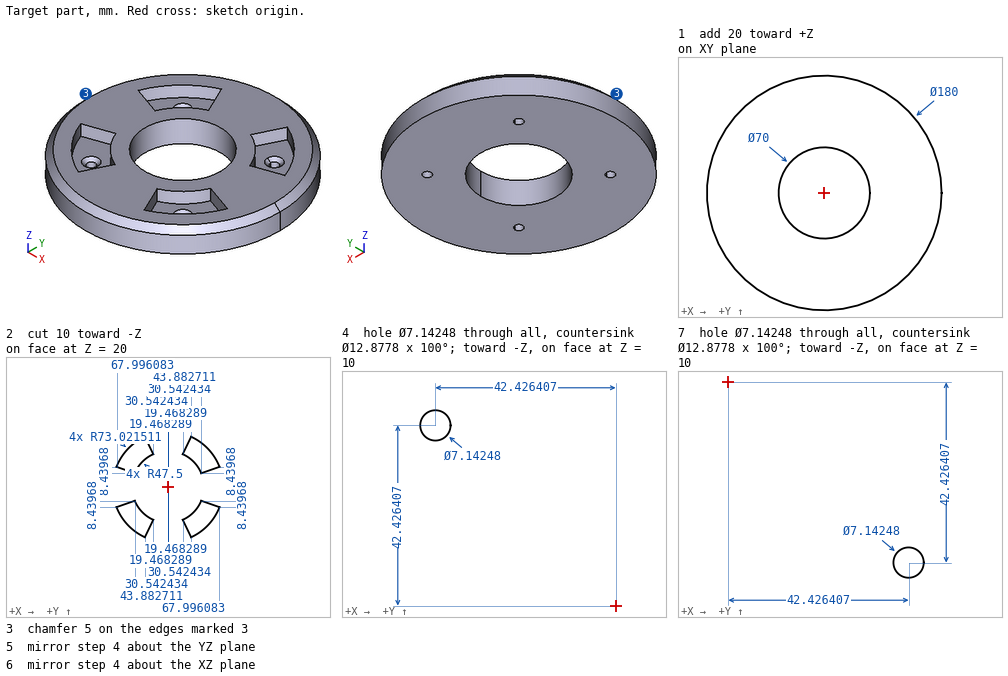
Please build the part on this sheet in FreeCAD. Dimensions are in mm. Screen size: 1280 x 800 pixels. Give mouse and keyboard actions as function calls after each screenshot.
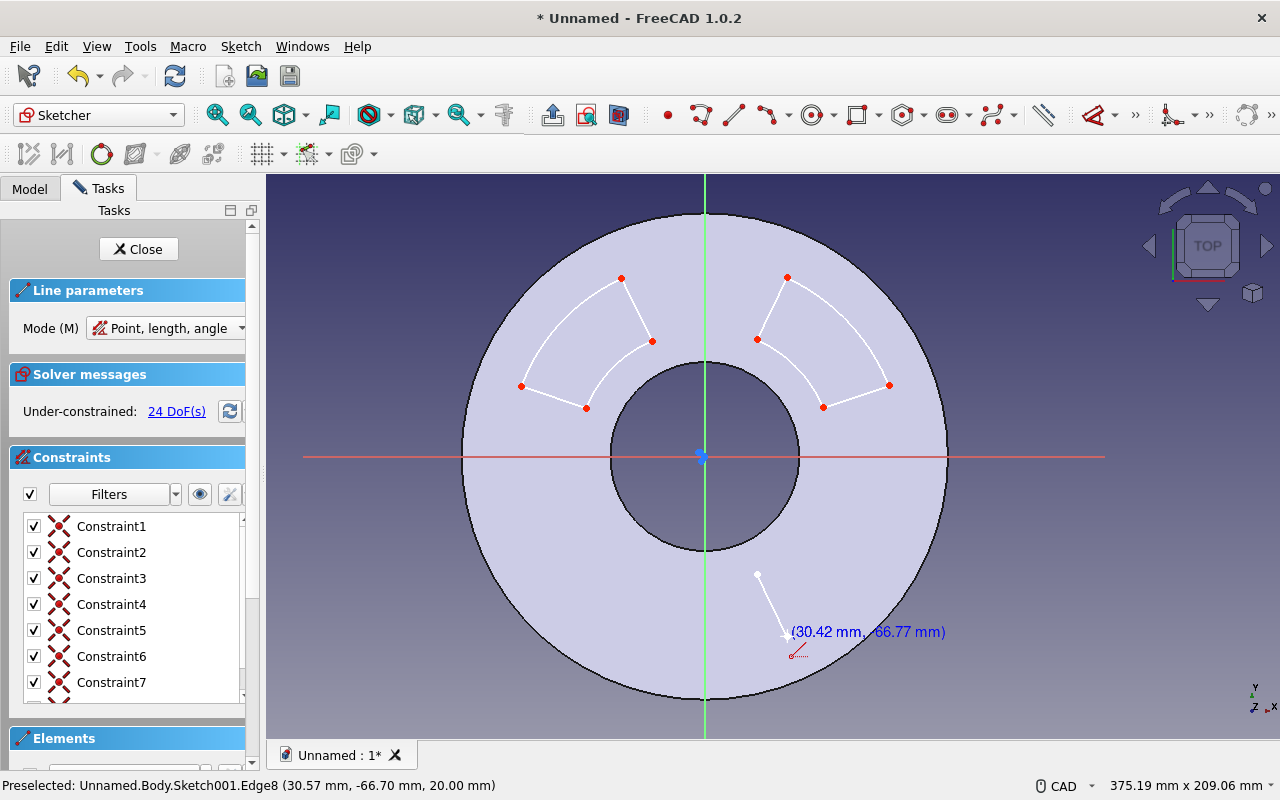
click(889, 528)
click(823, 506)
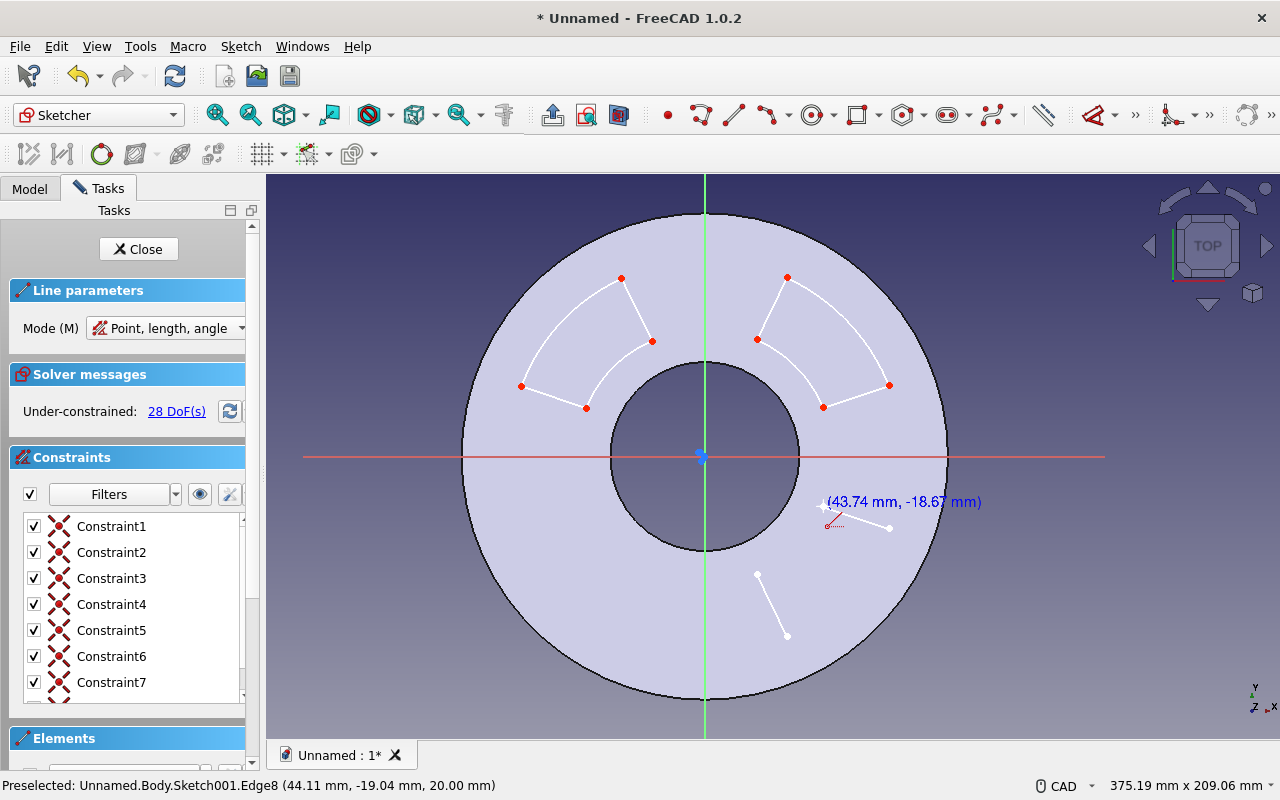
click(766, 116)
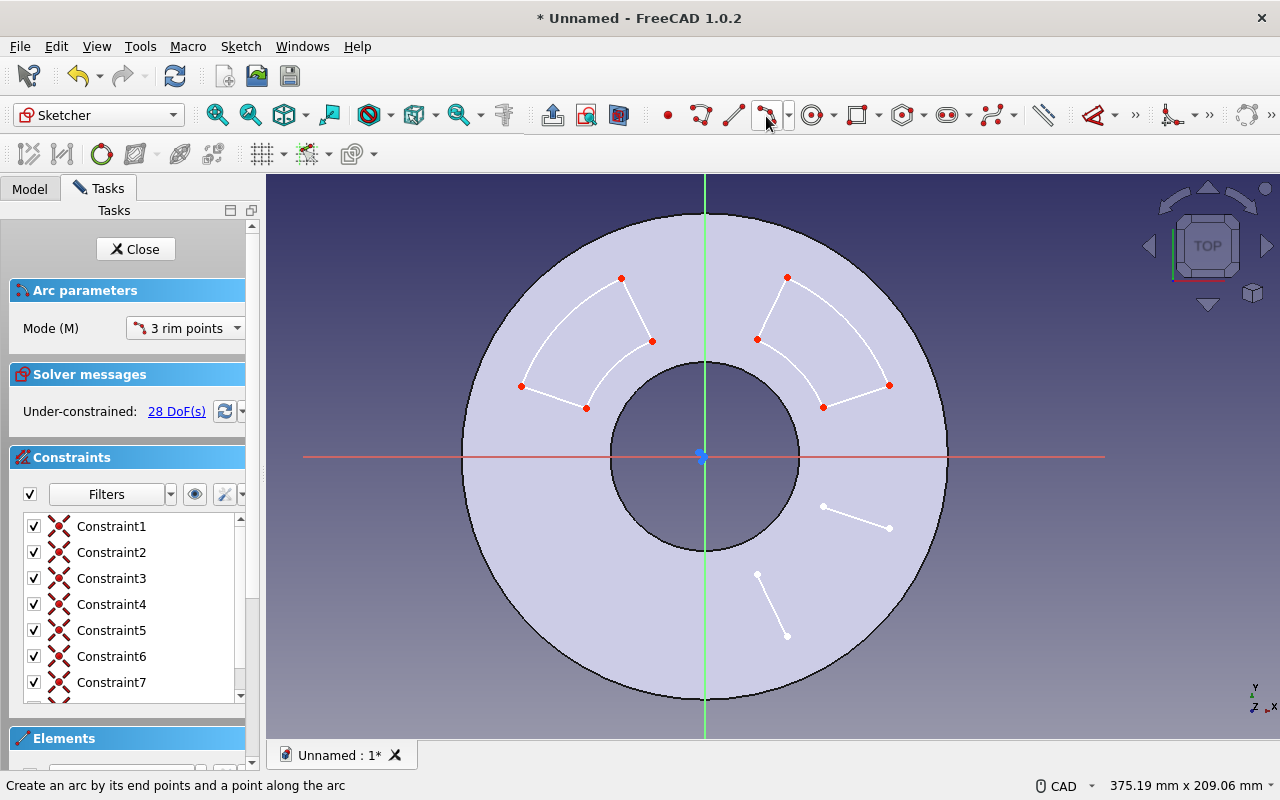
click(787, 637)
click(889, 529)
click(848, 592)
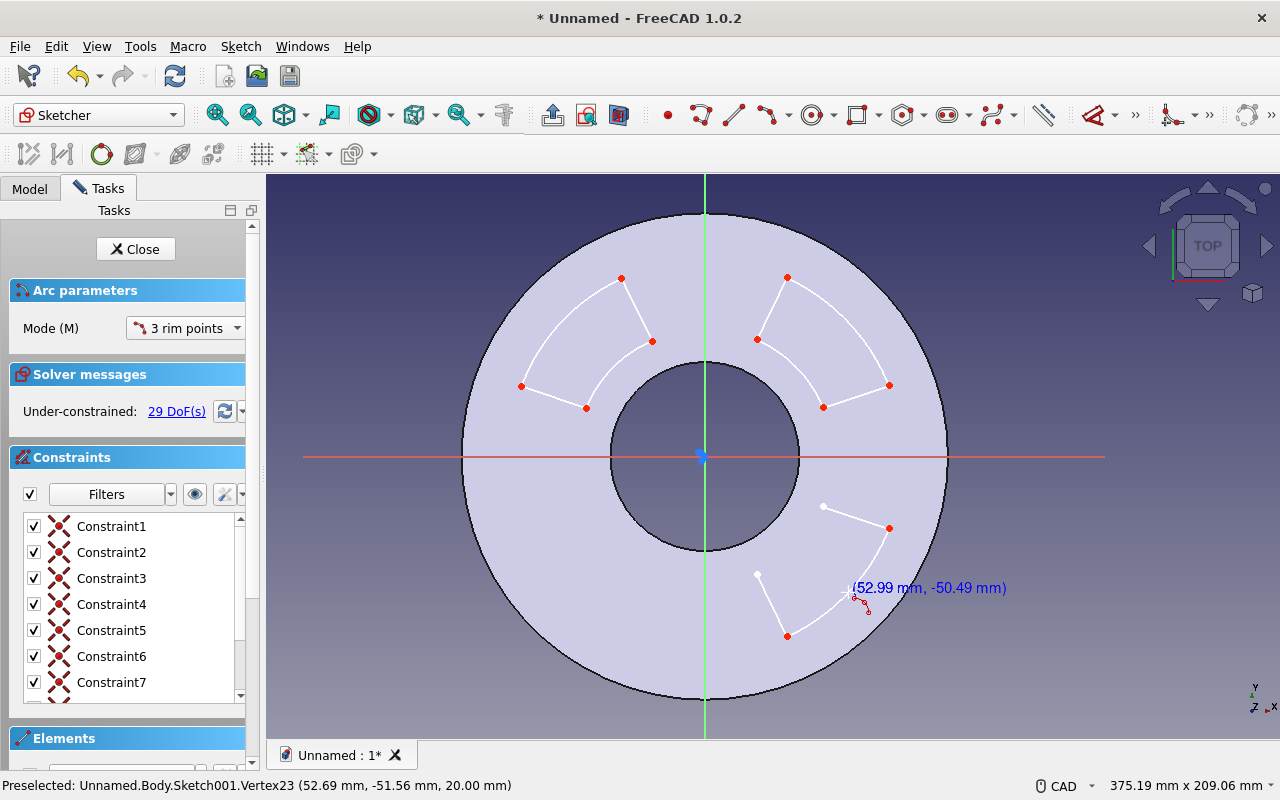
click(823, 507)
click(757, 575)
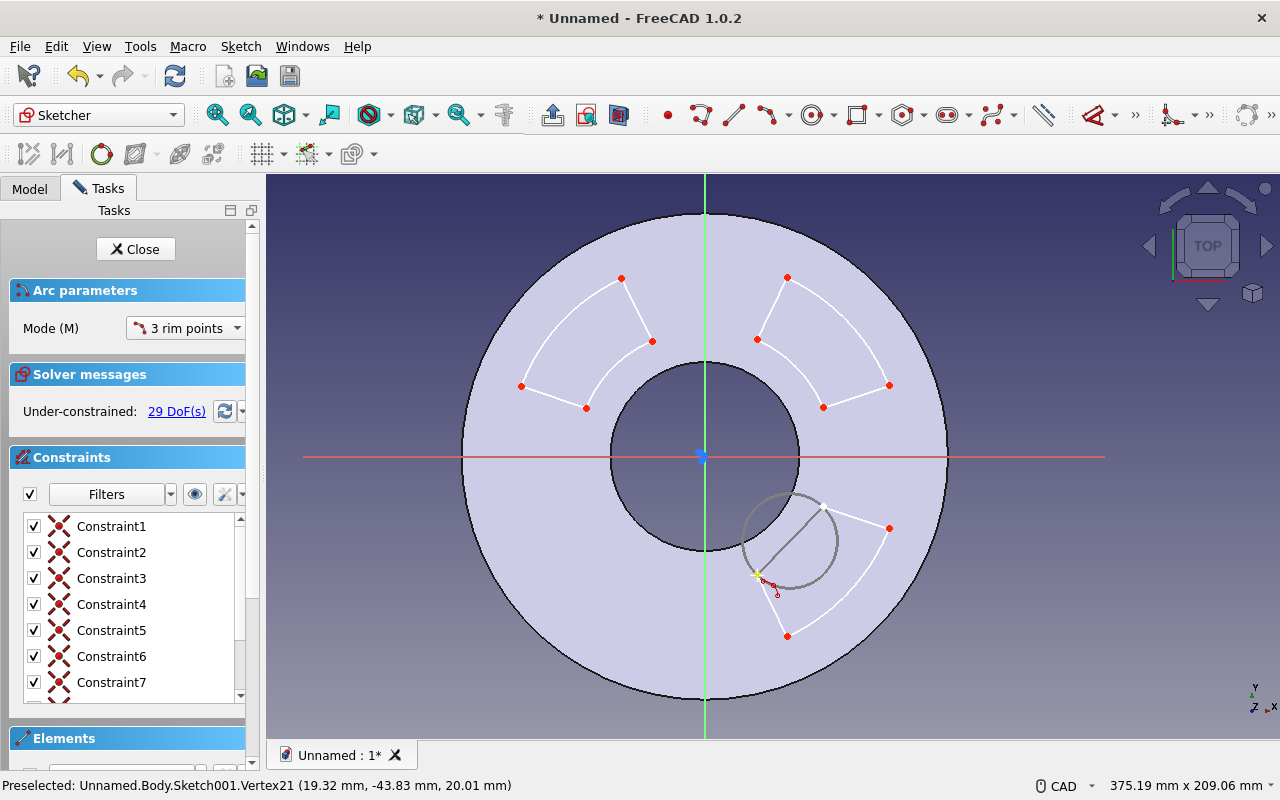
scroll(797, 546, up, 3)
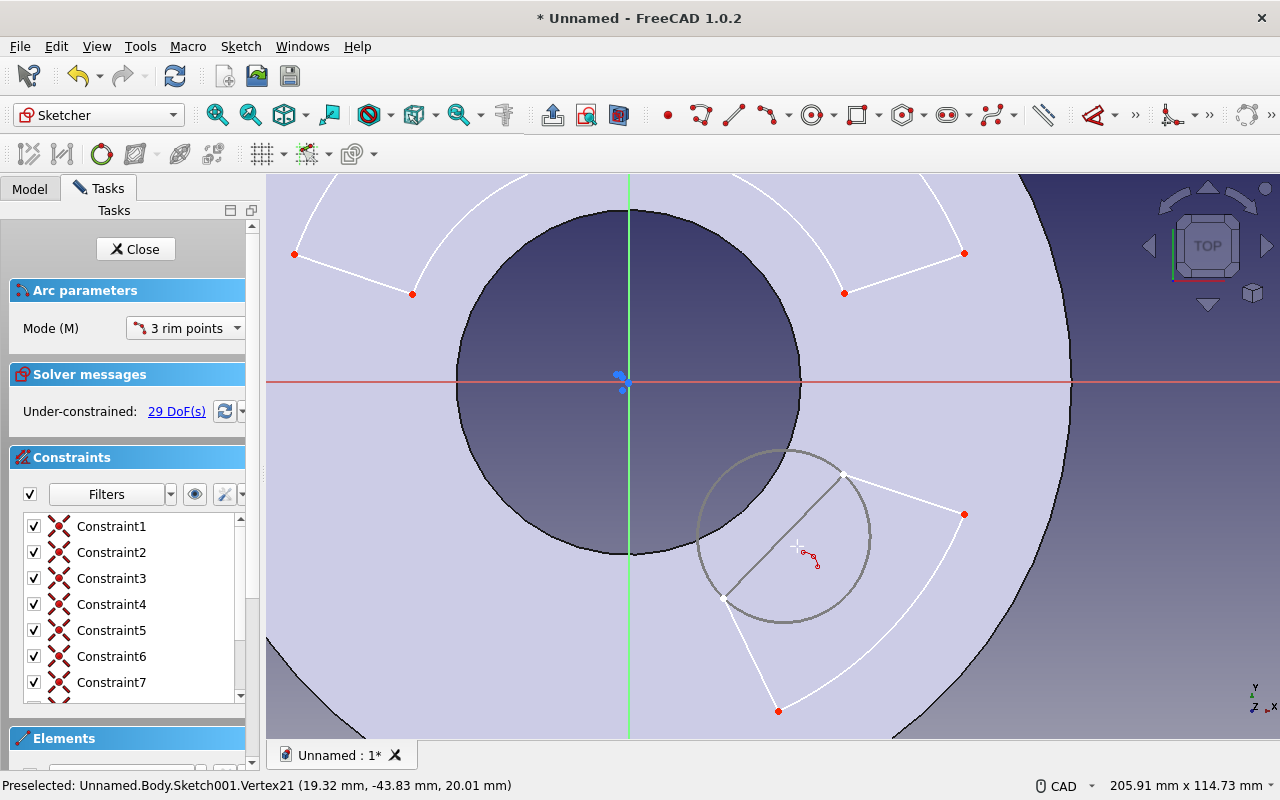
click(796, 545)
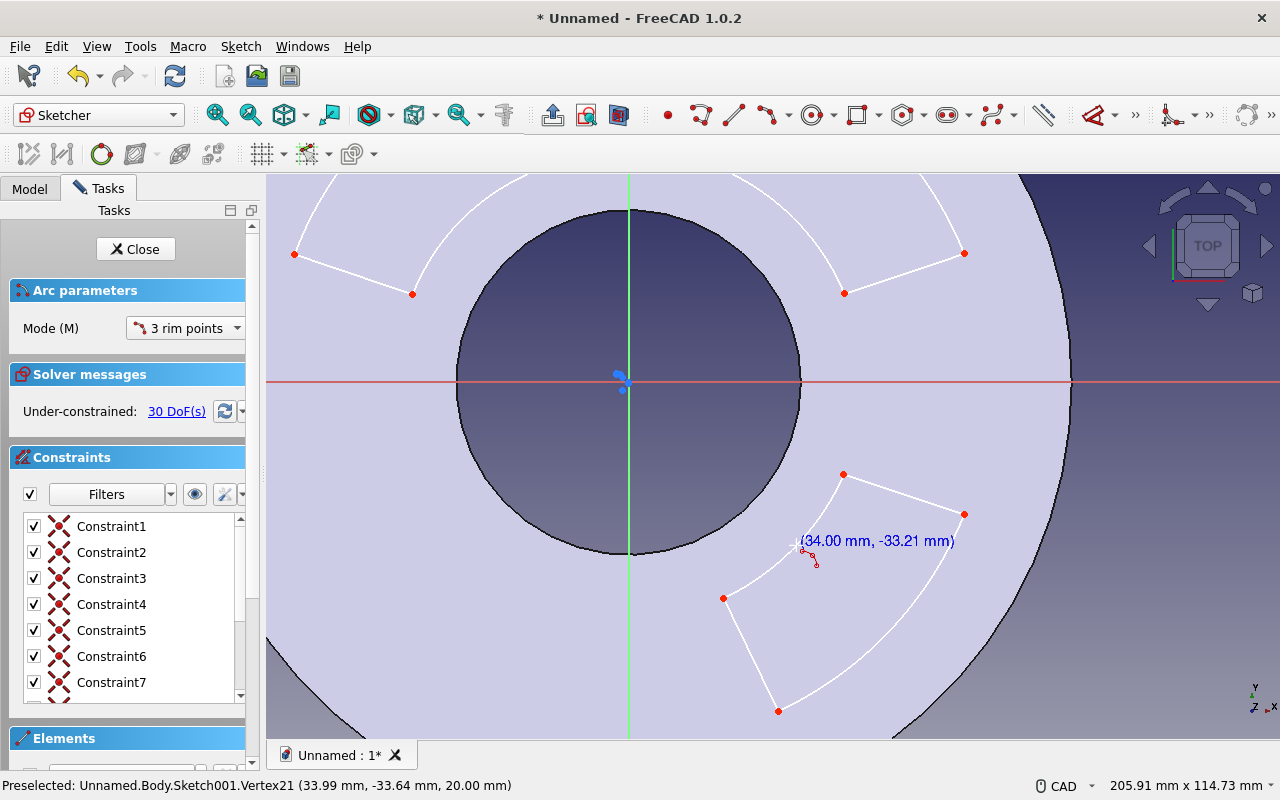
click(734, 116)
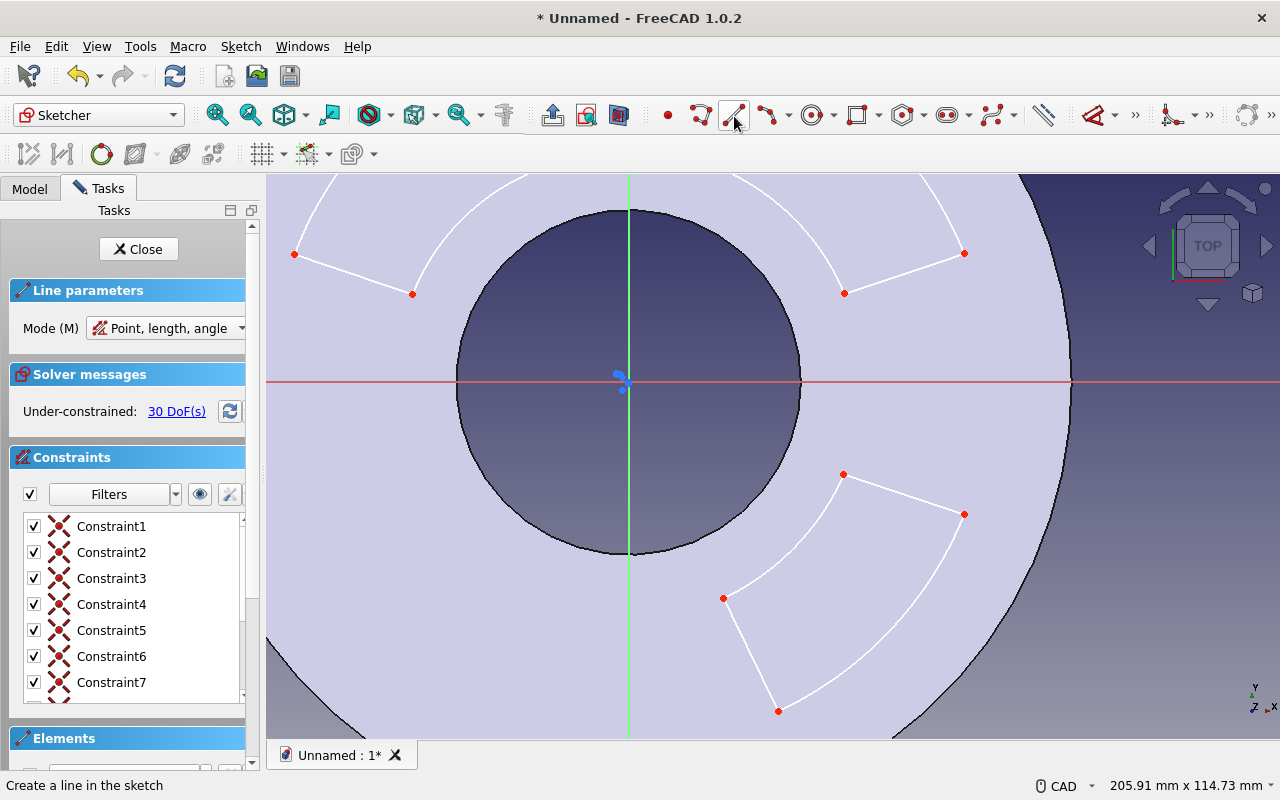
click(412, 472)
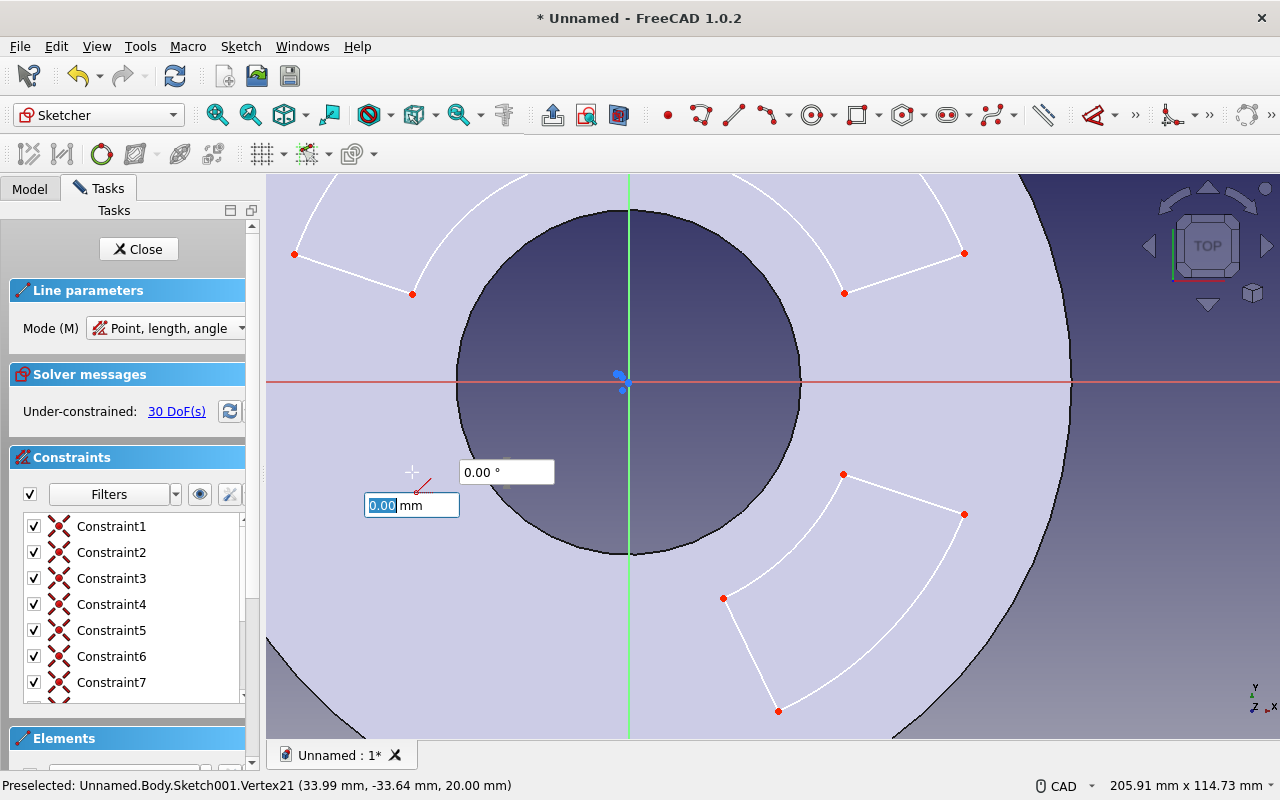
scroll(797, 547, down, 3)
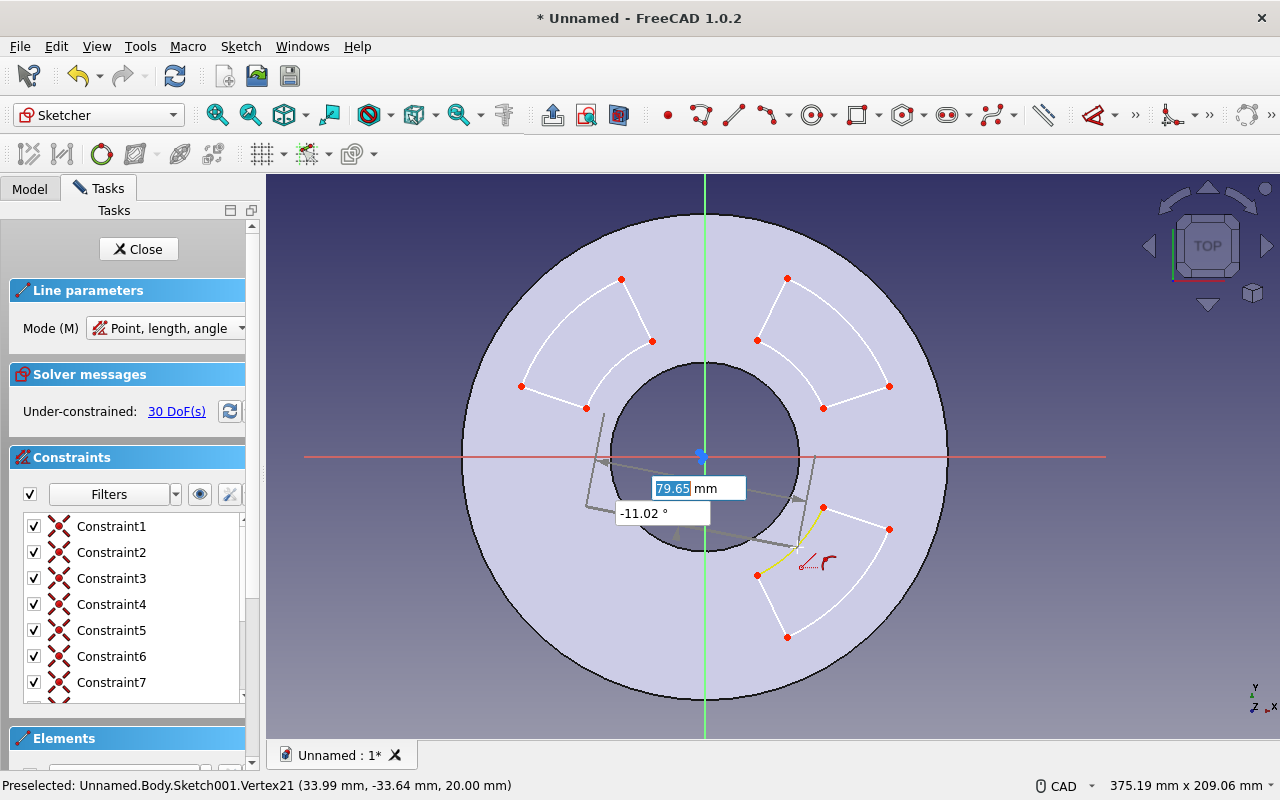
click(521, 529)